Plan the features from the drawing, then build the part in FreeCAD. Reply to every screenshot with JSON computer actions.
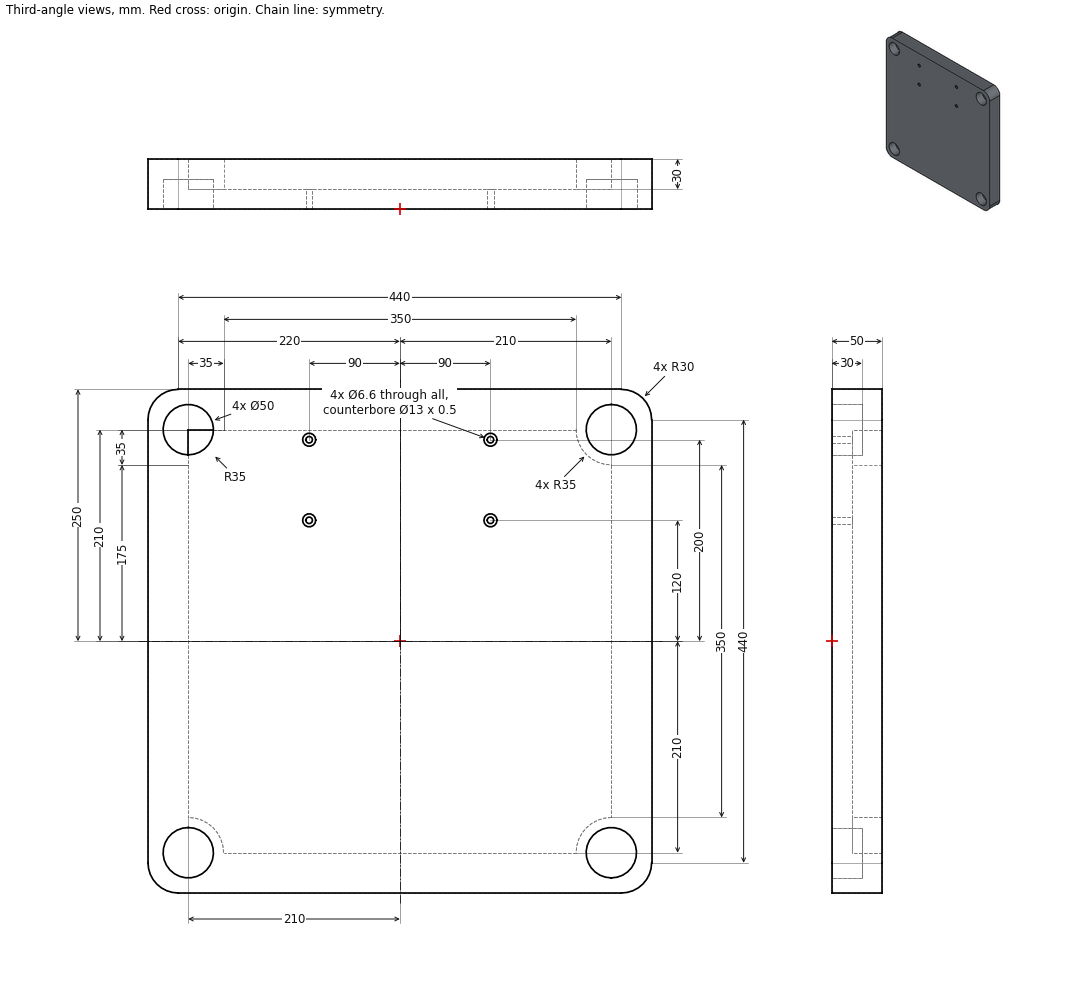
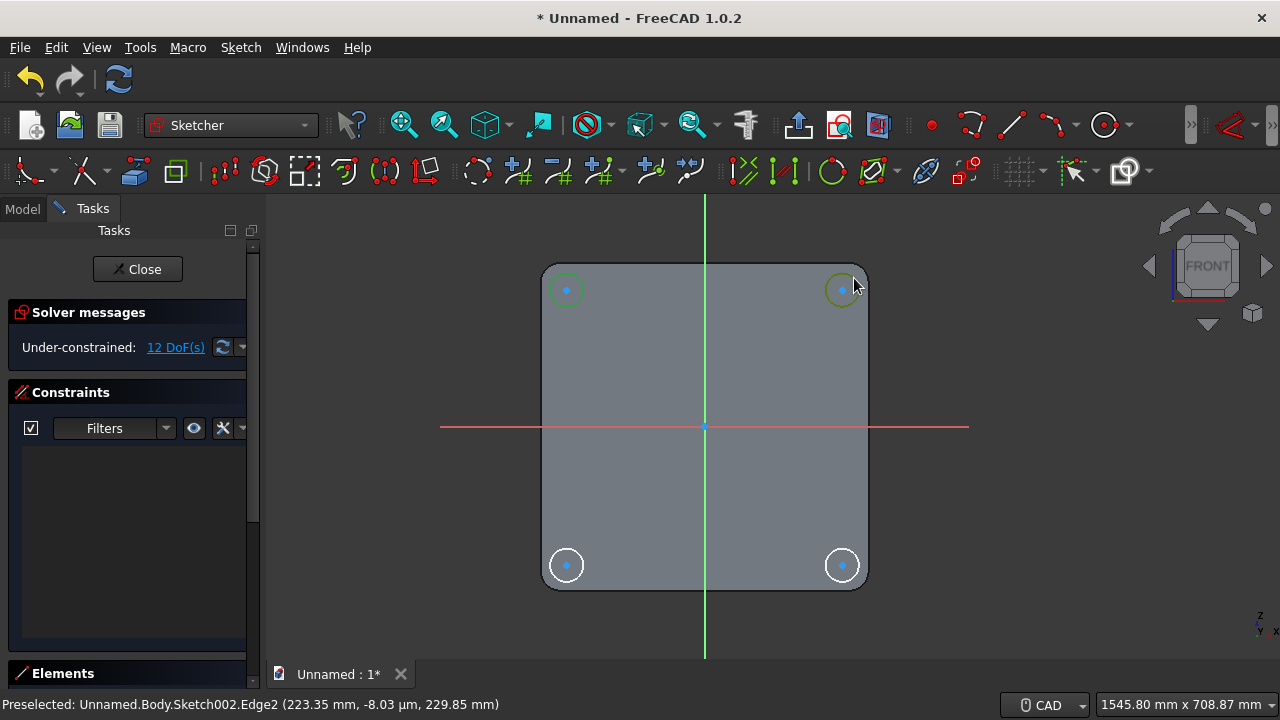
{"action": "left_click", "coordinate": [854, 553]}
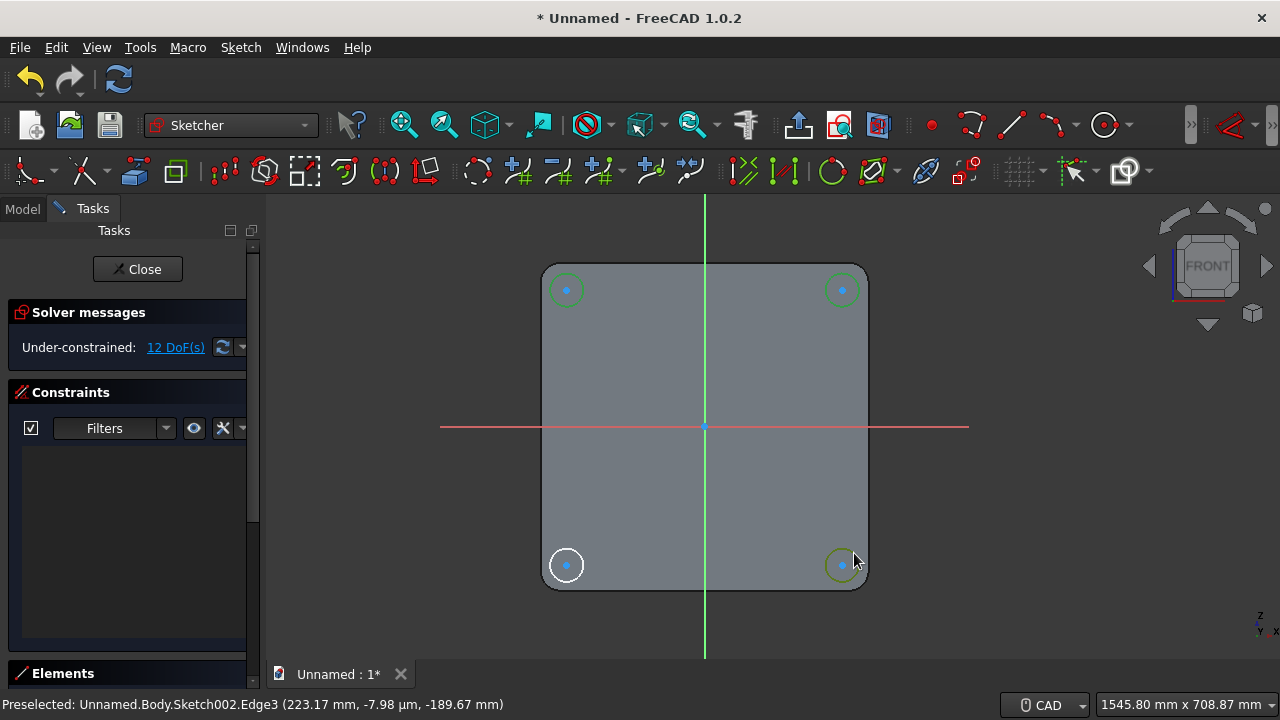
{"action": "left_click", "coordinate": [578, 553]}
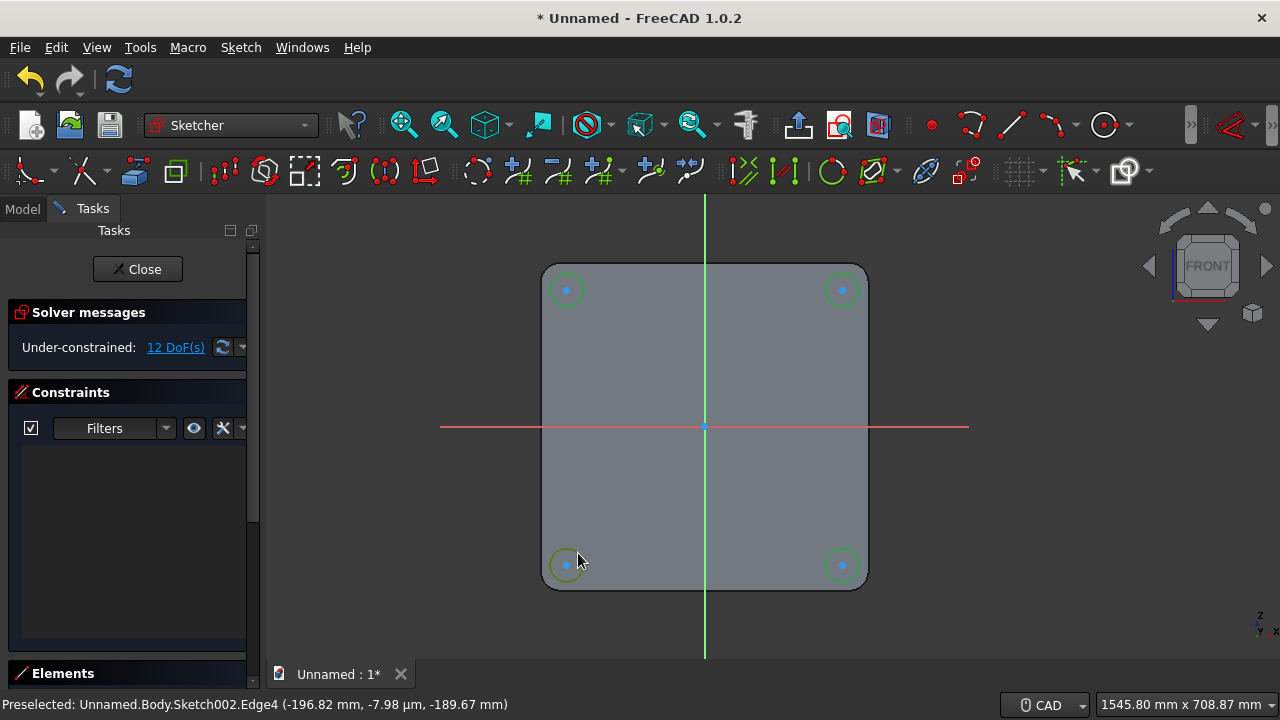
{"action": "key", "text": "e"}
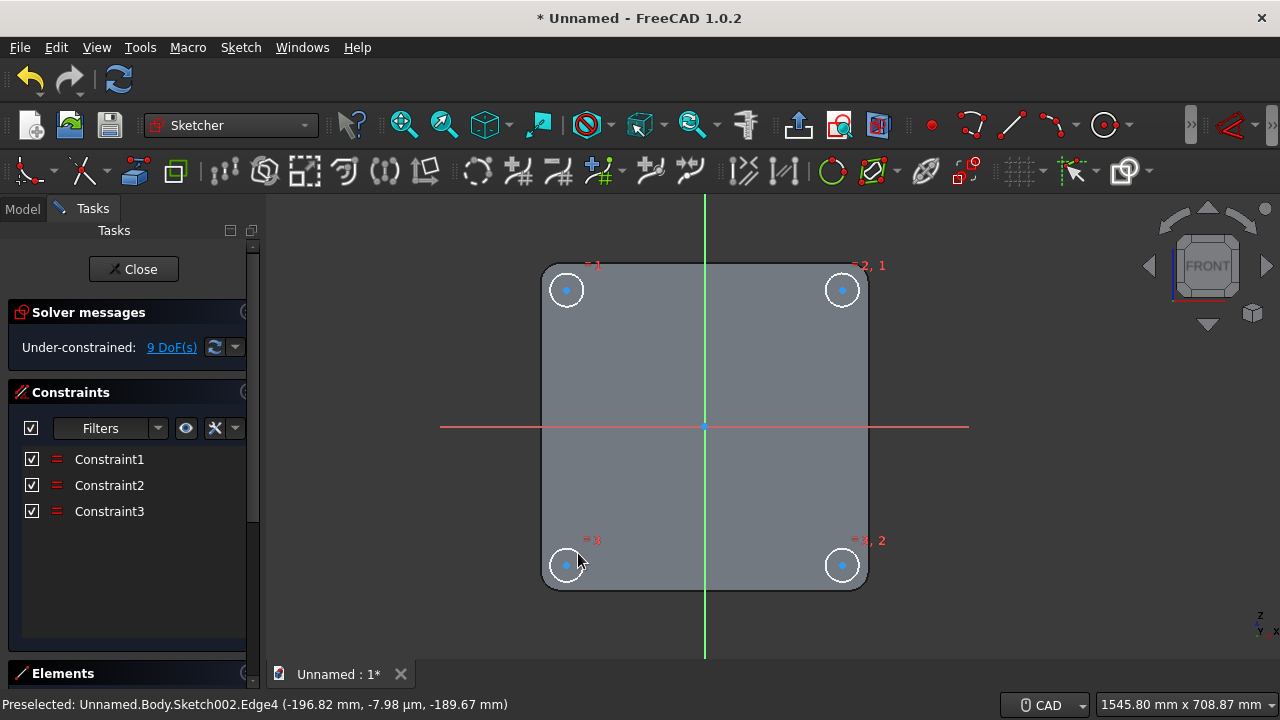
{"action": "left_click", "coordinate": [567, 290]}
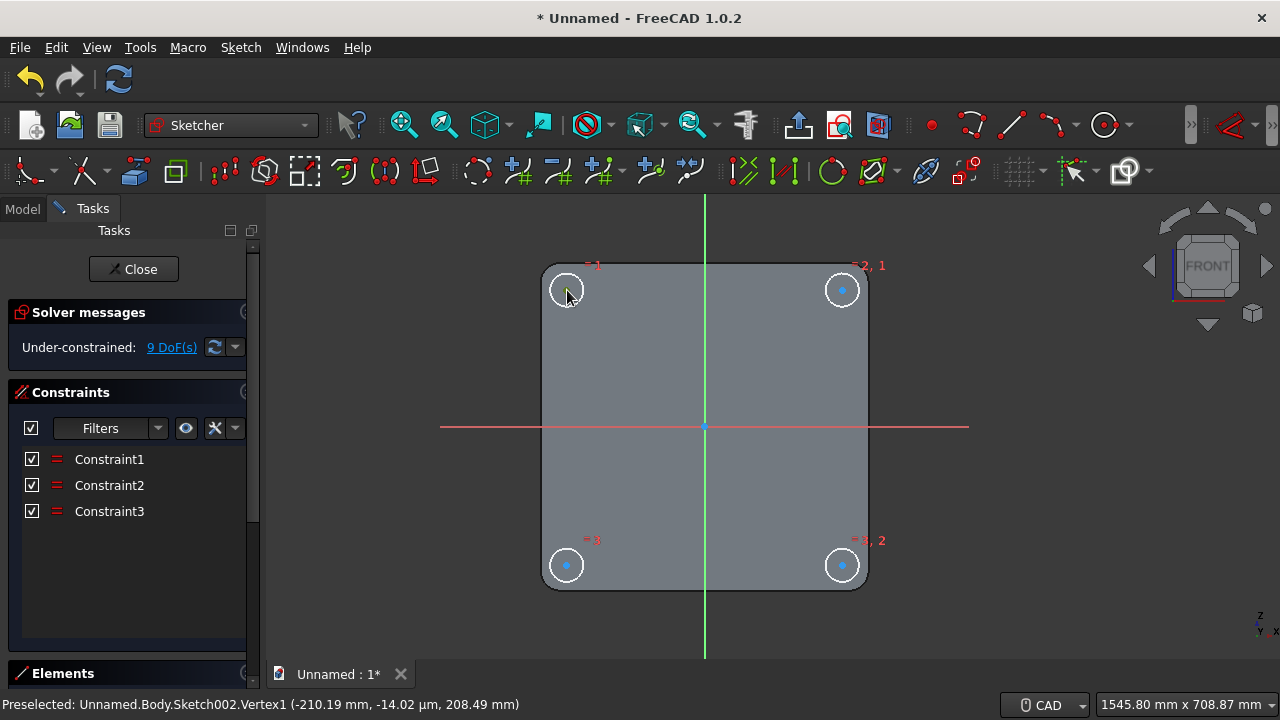
{"action": "left_click", "coordinate": [842, 290]}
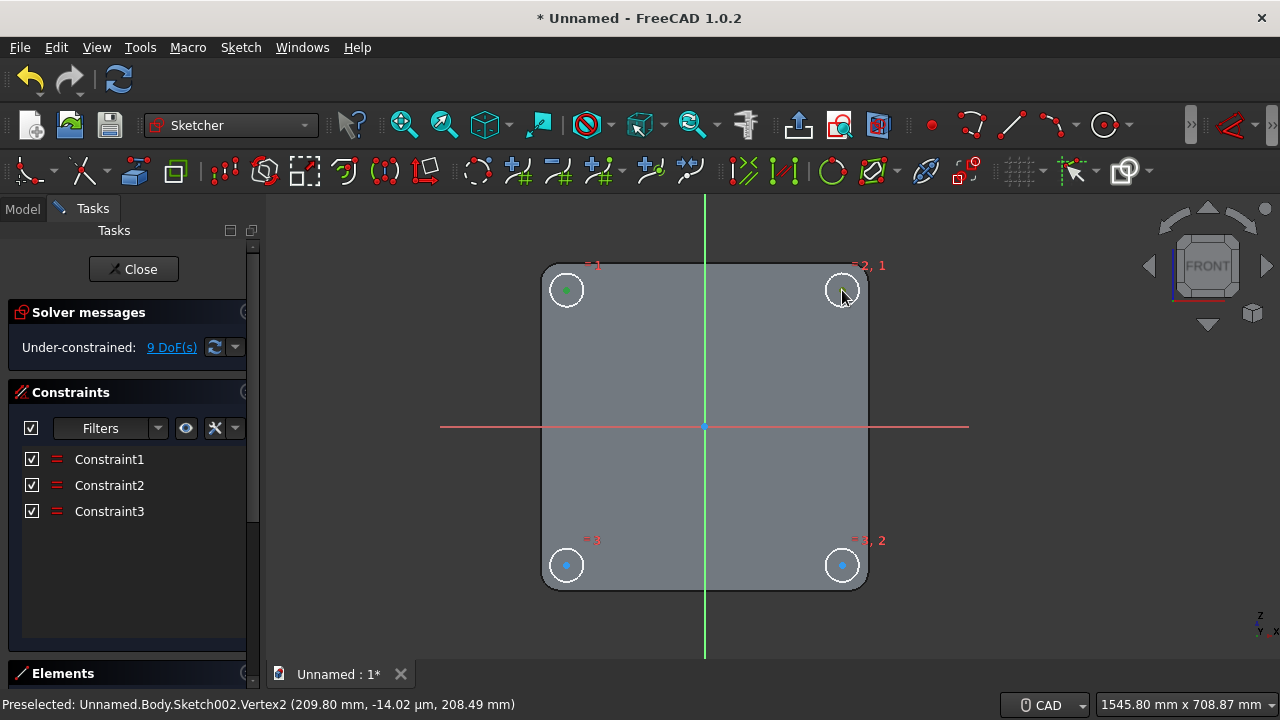
{"action": "key", "text": "h"}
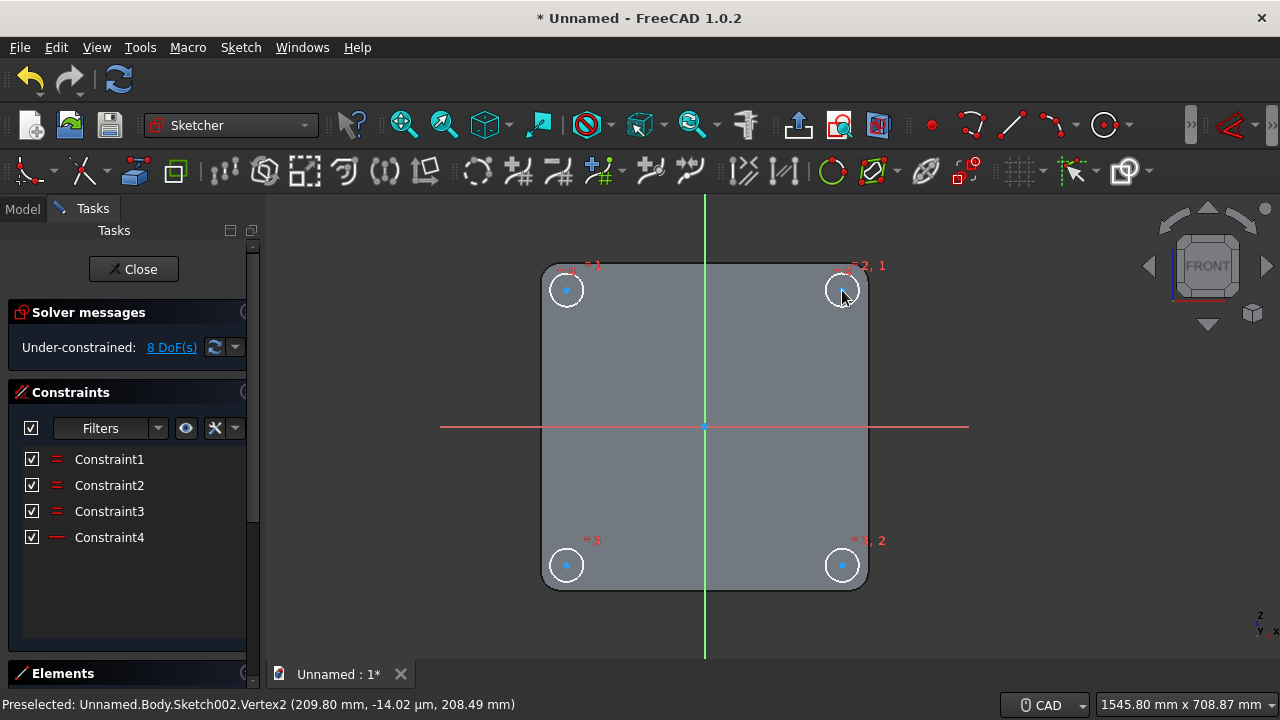
{"action": "left_click", "coordinate": [842, 290]}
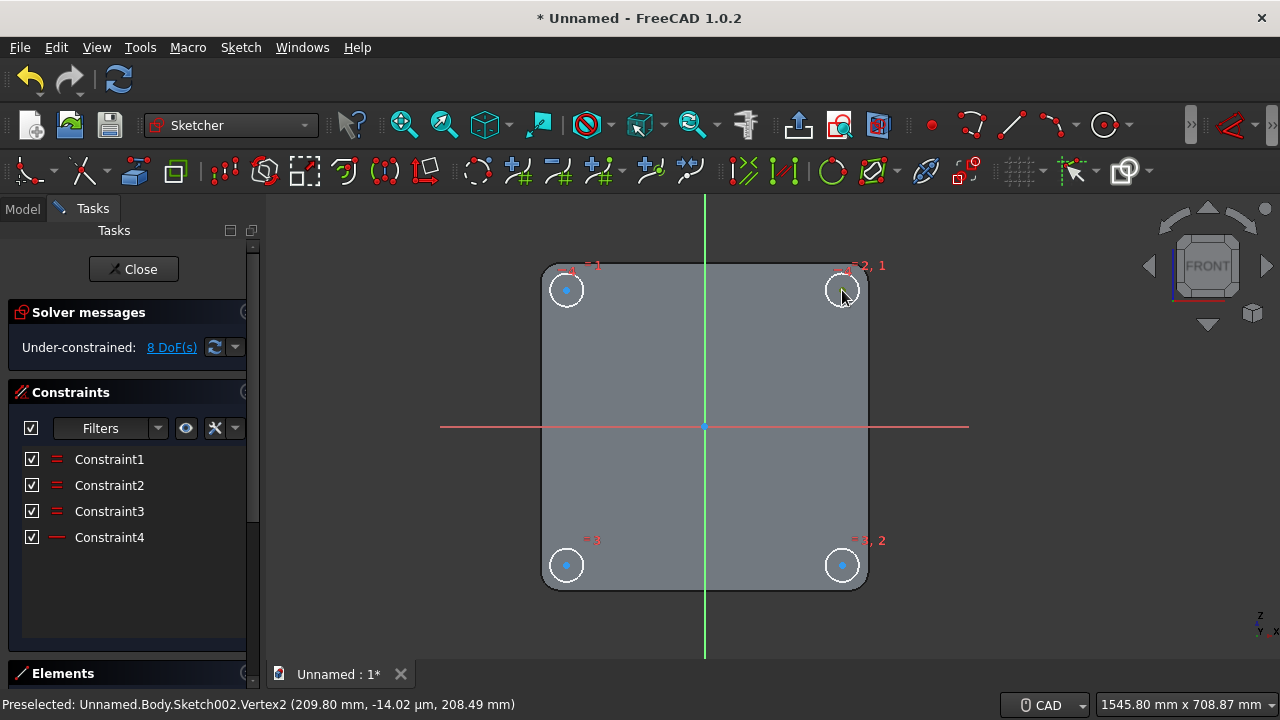
{"action": "left_click", "coordinate": [842, 565]}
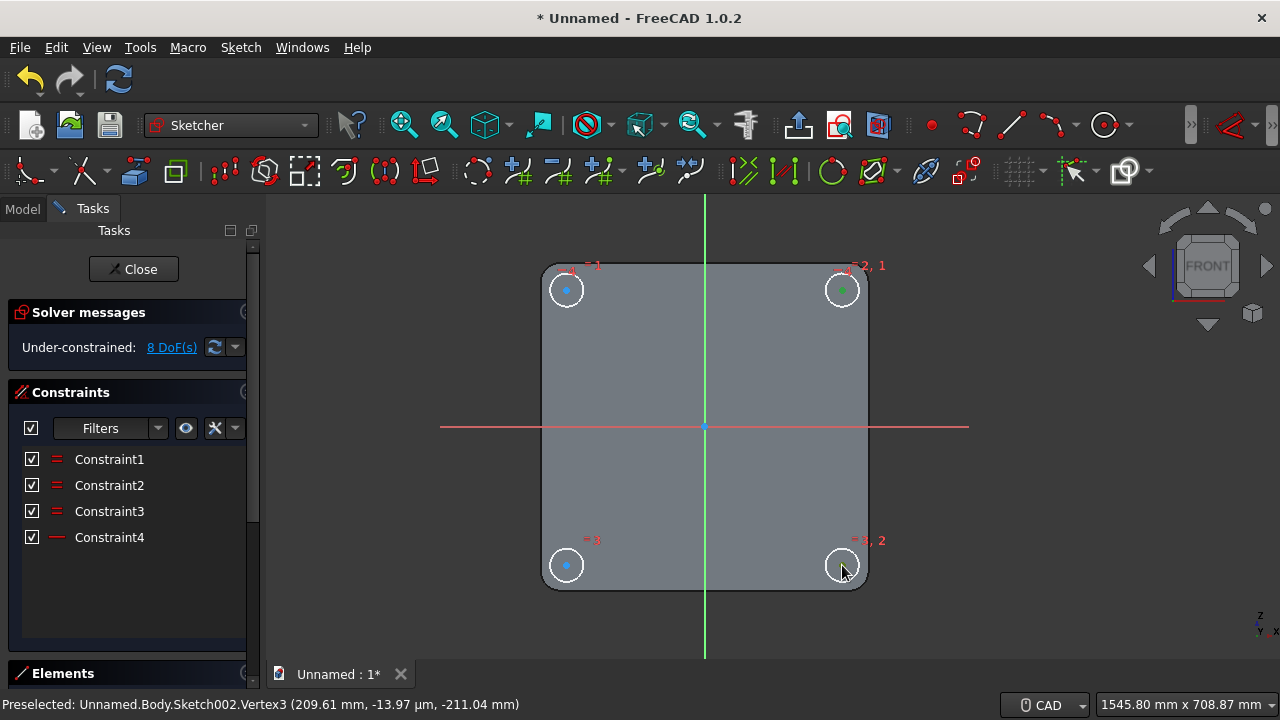
{"action": "key", "text": "v"}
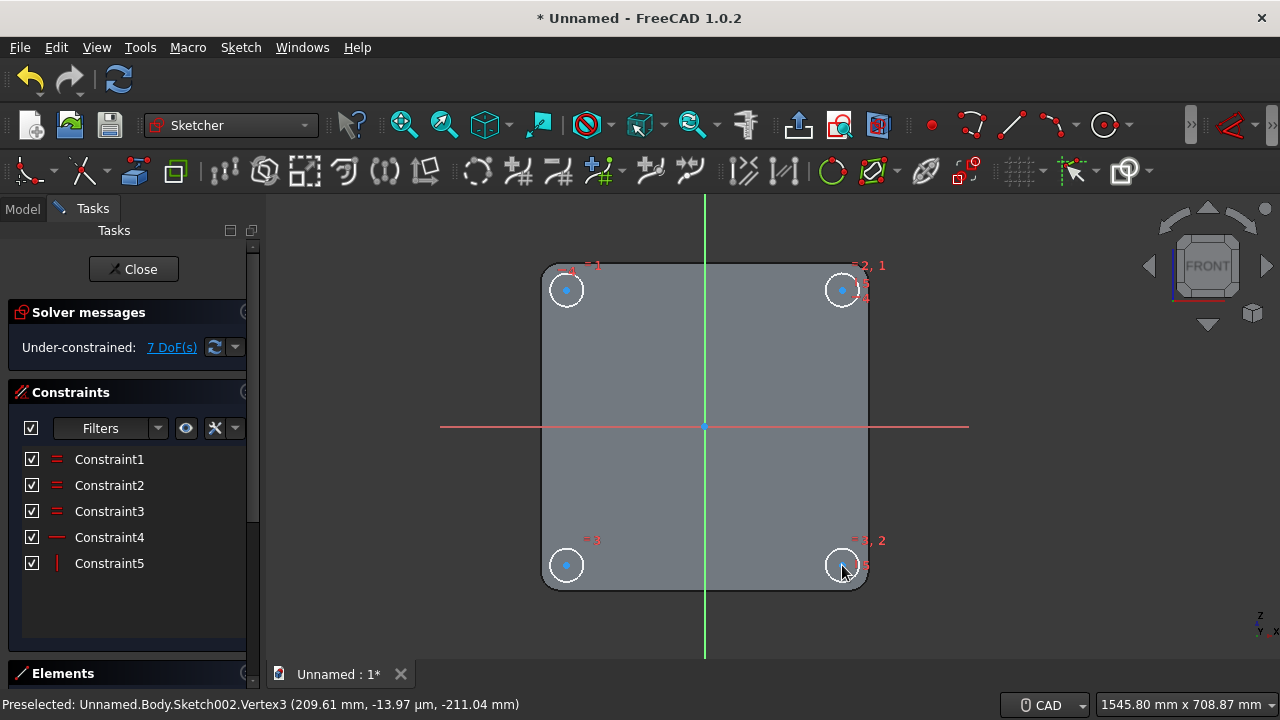
{"action": "left_click", "coordinate": [567, 290]}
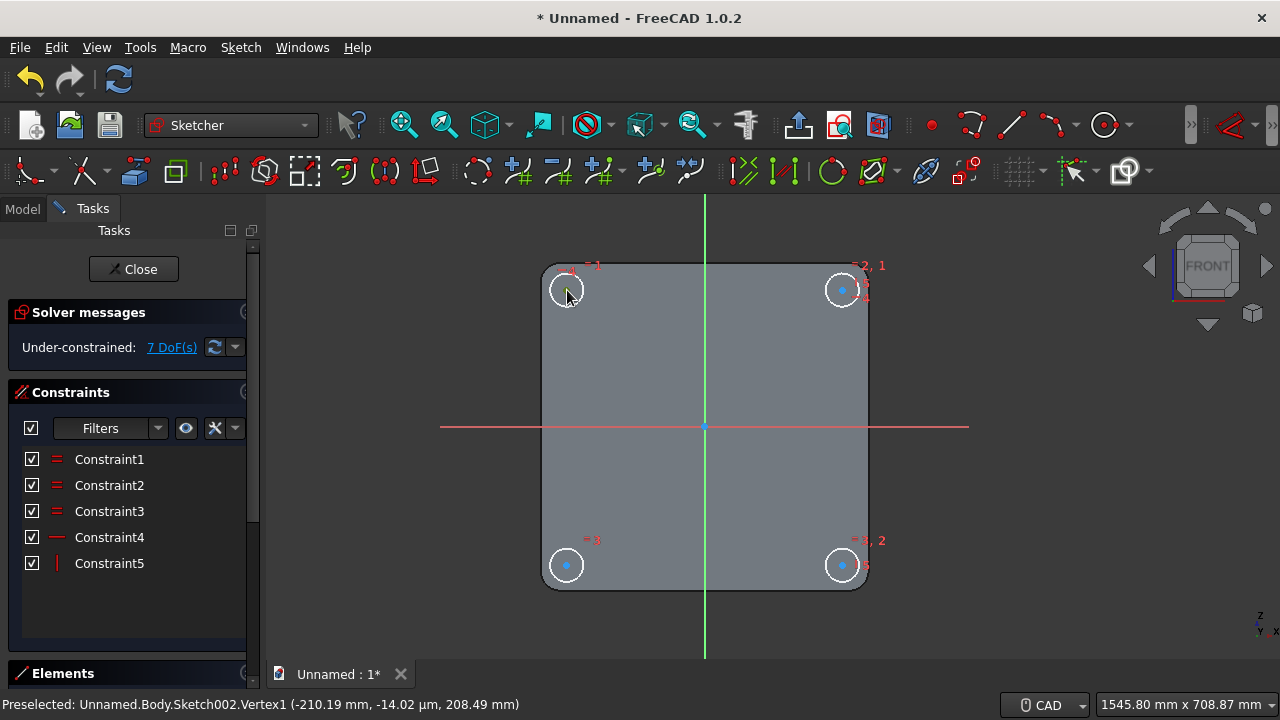
{"action": "left_click", "coordinate": [567, 565]}